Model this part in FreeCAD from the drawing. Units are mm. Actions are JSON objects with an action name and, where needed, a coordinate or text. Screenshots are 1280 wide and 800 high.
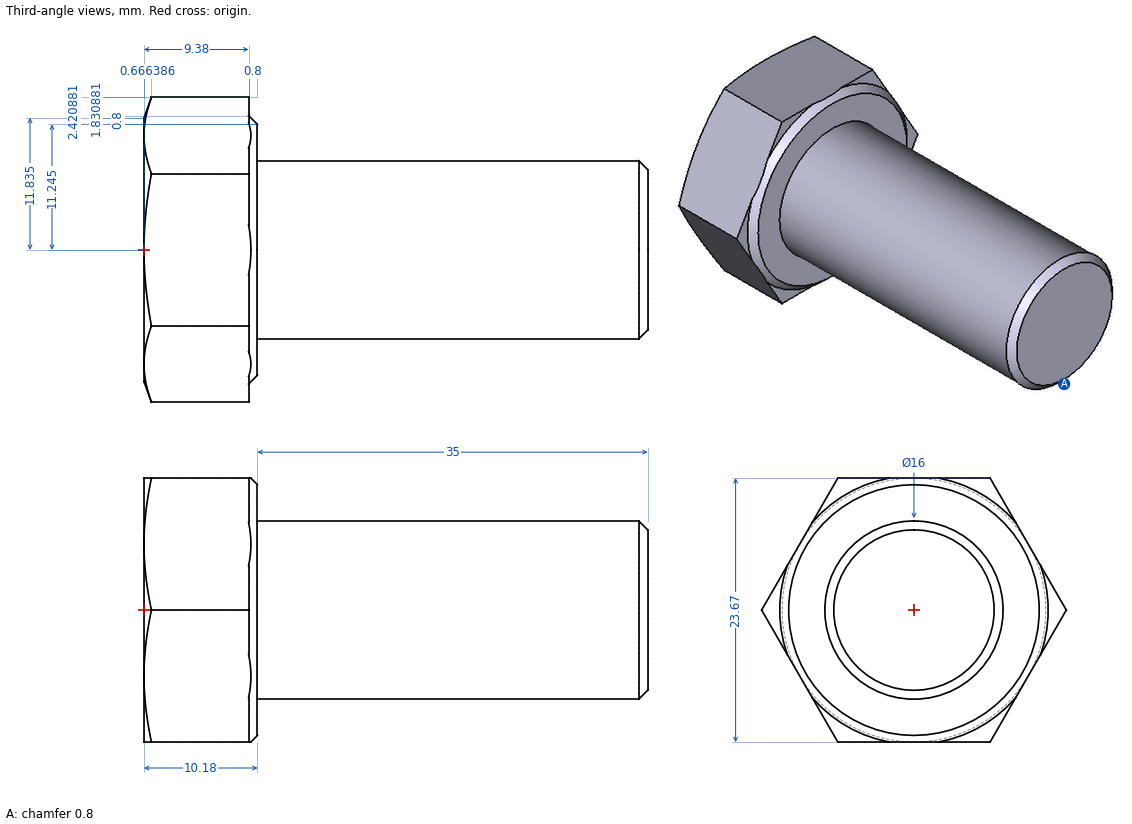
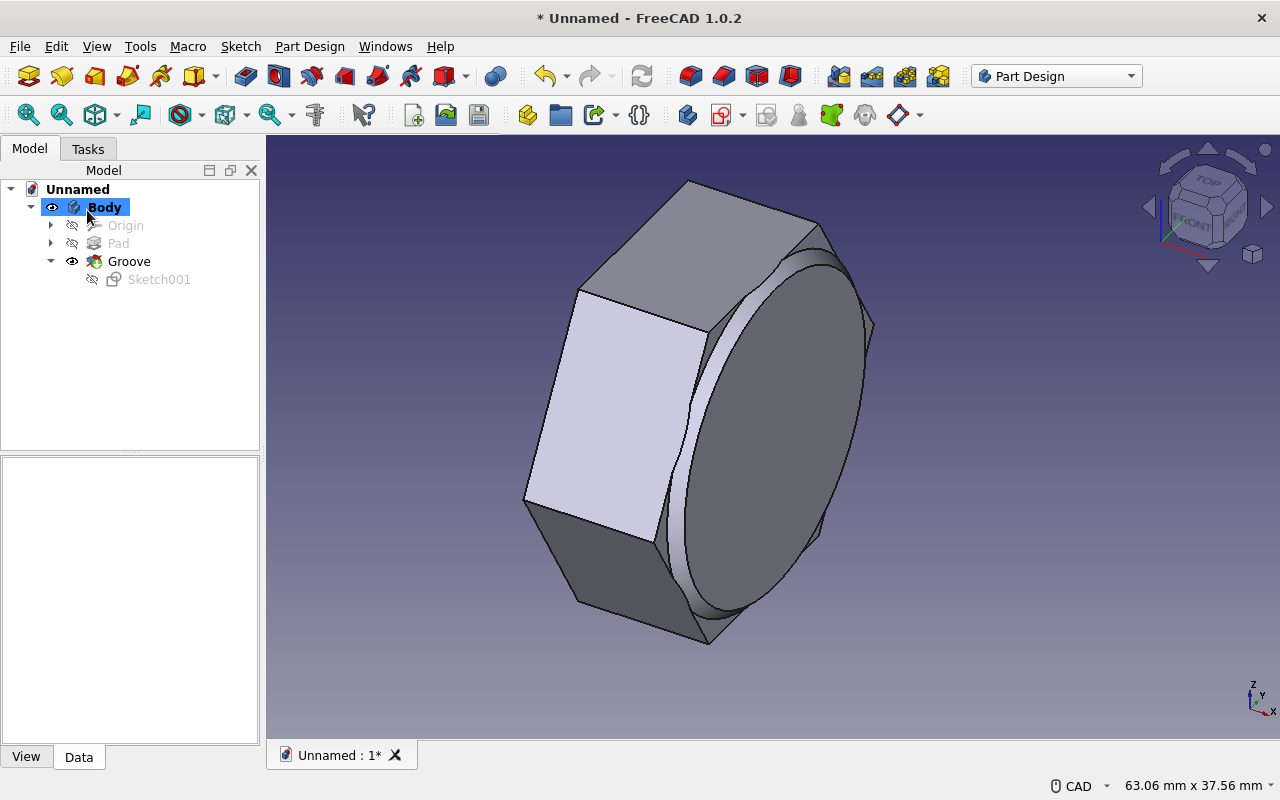
{"action": "key", "text": "v f"}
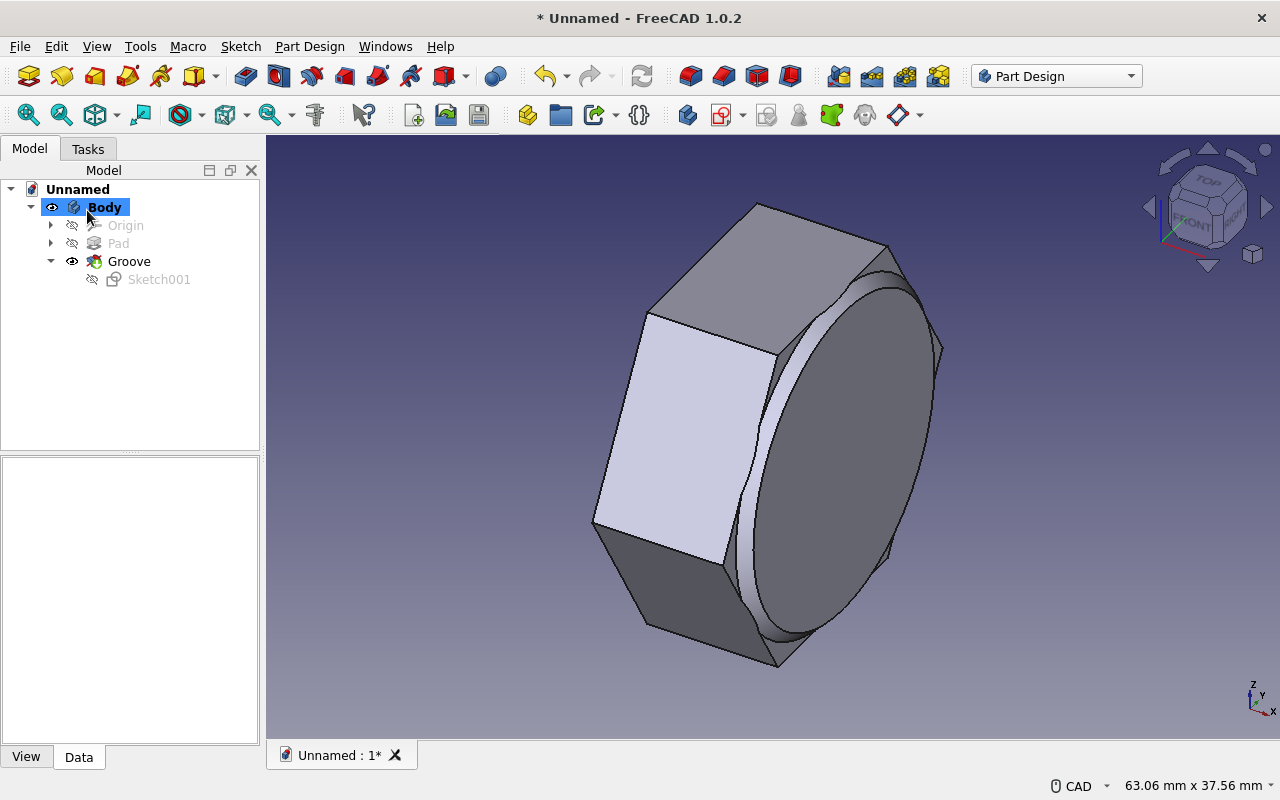
{"action": "left_click", "coordinate": [720, 116]}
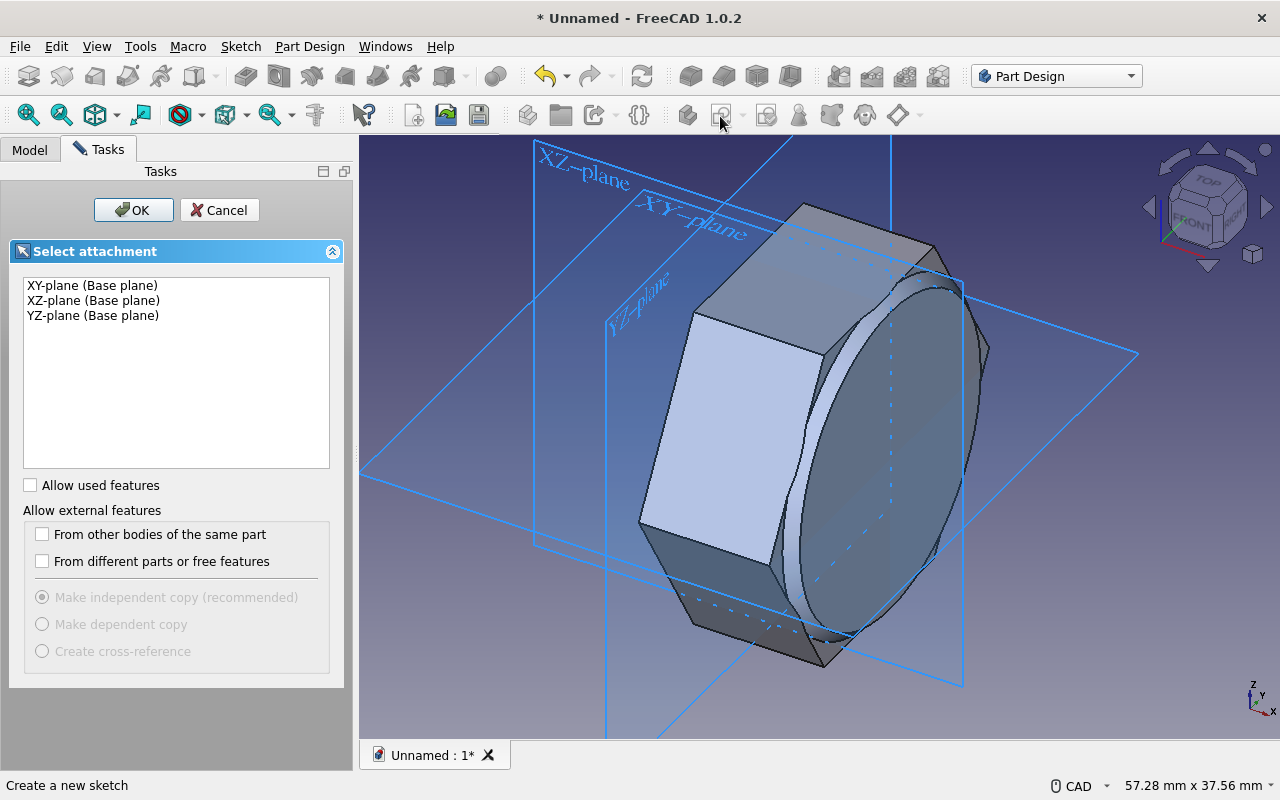
{"action": "left_click", "coordinate": [84, 286]}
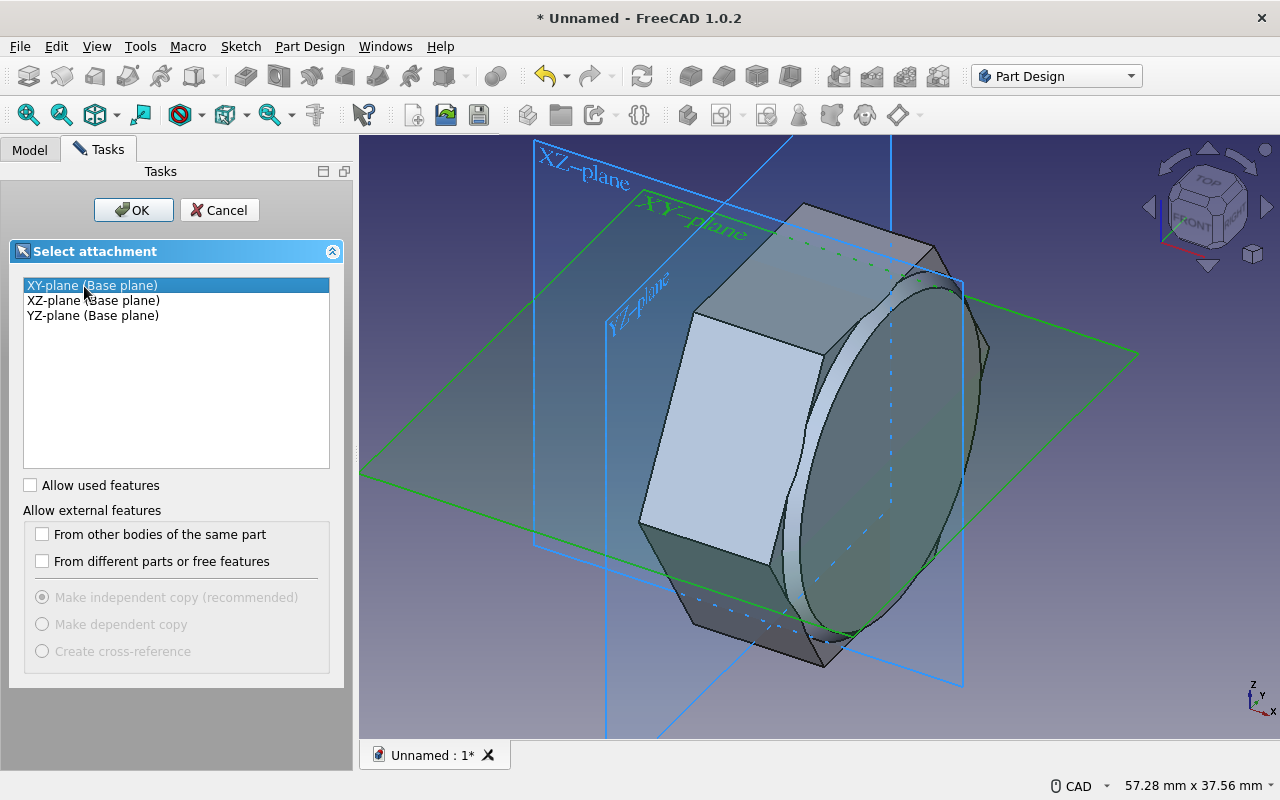
{"action": "left_click", "coordinate": [134, 210]}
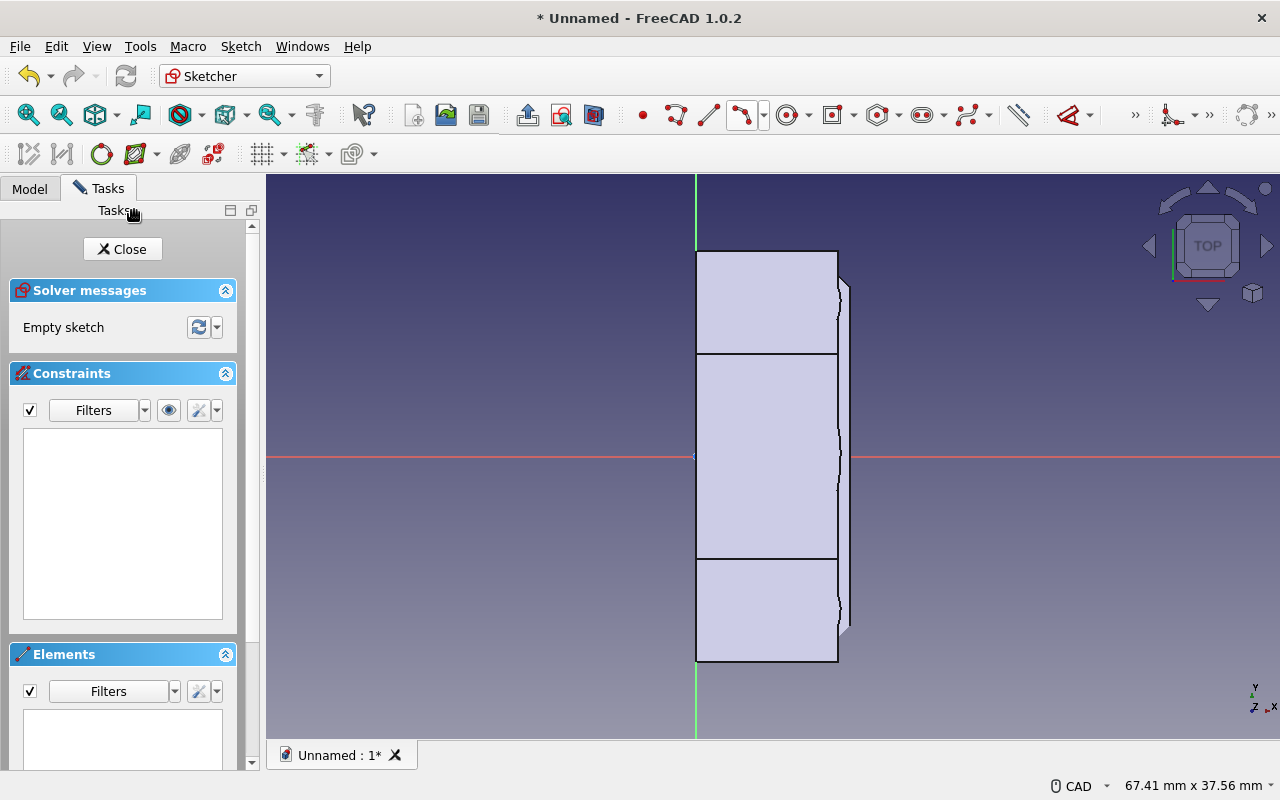
{"action": "left_click", "coordinate": [594, 116]}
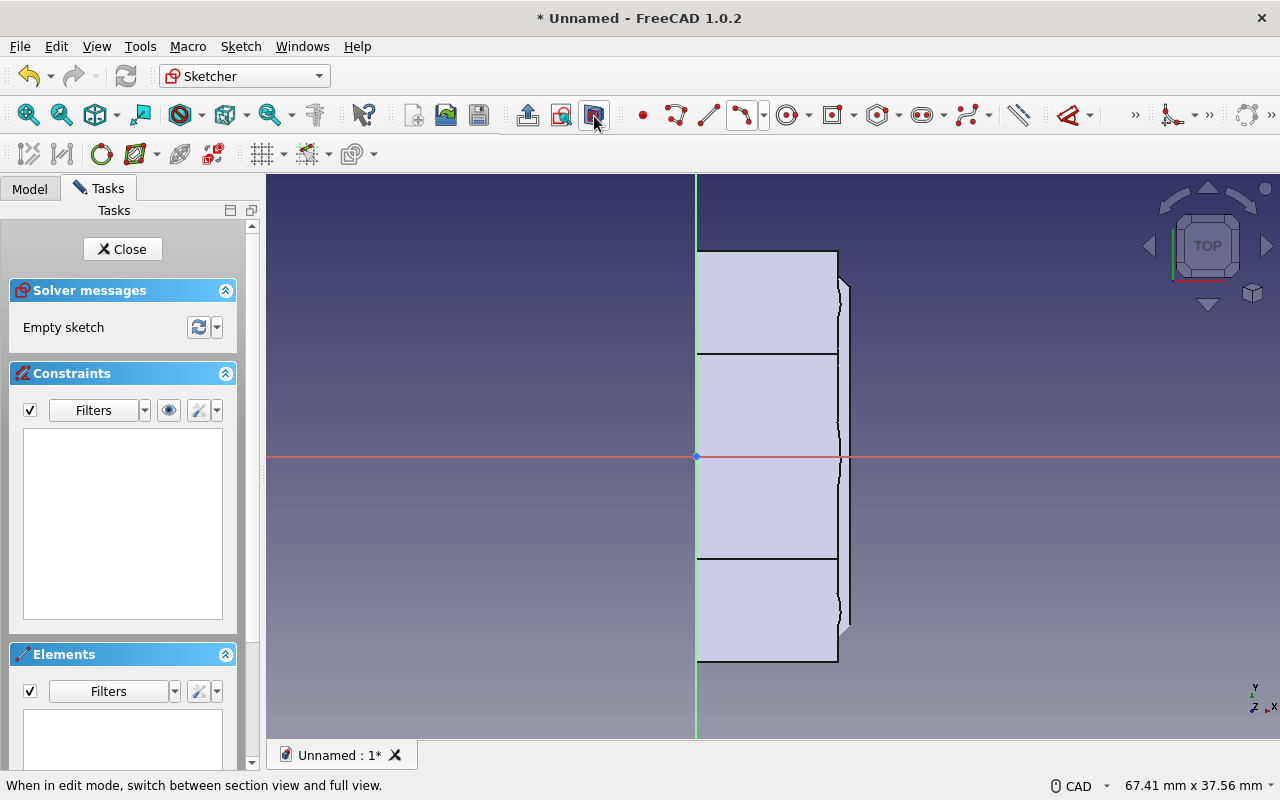
{"action": "scroll", "coordinate": [701, 249], "scroll_direction": "up", "scroll_amount": 13}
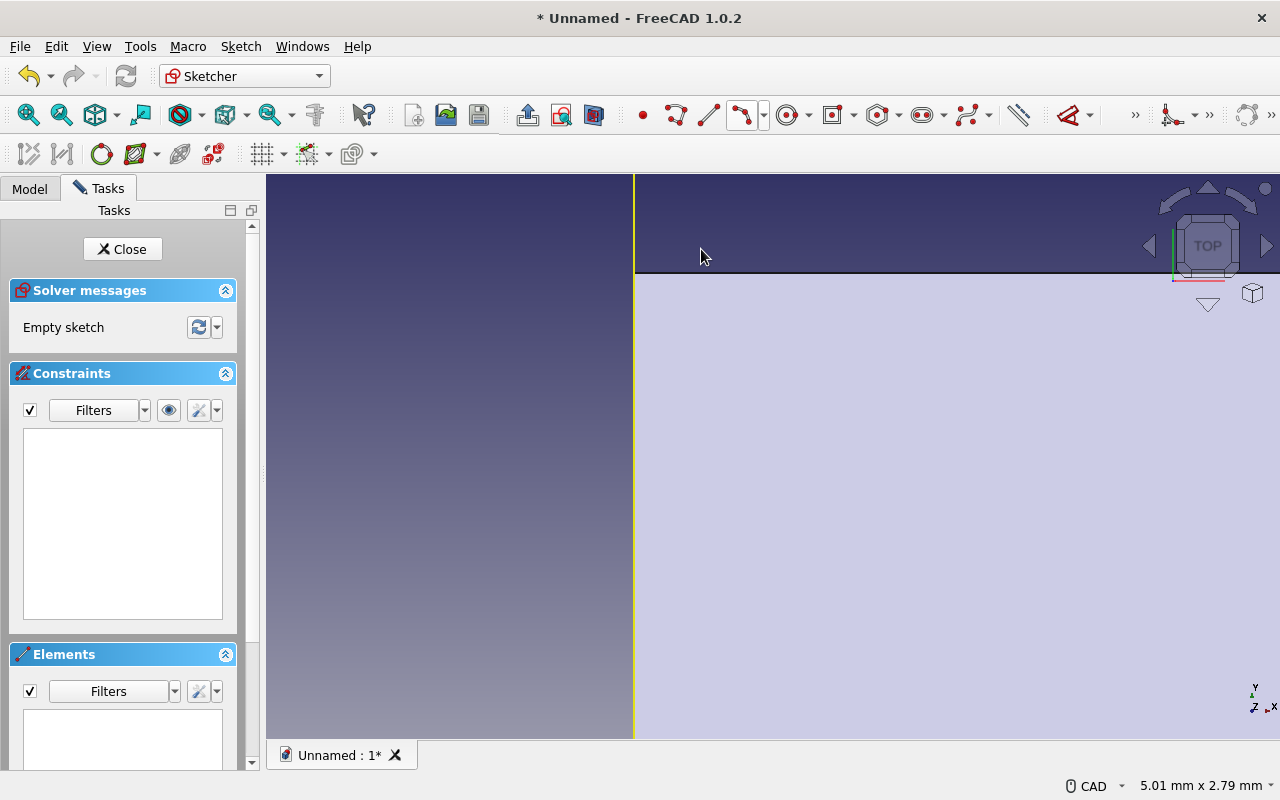
{"action": "left_click", "coordinate": [676, 116]}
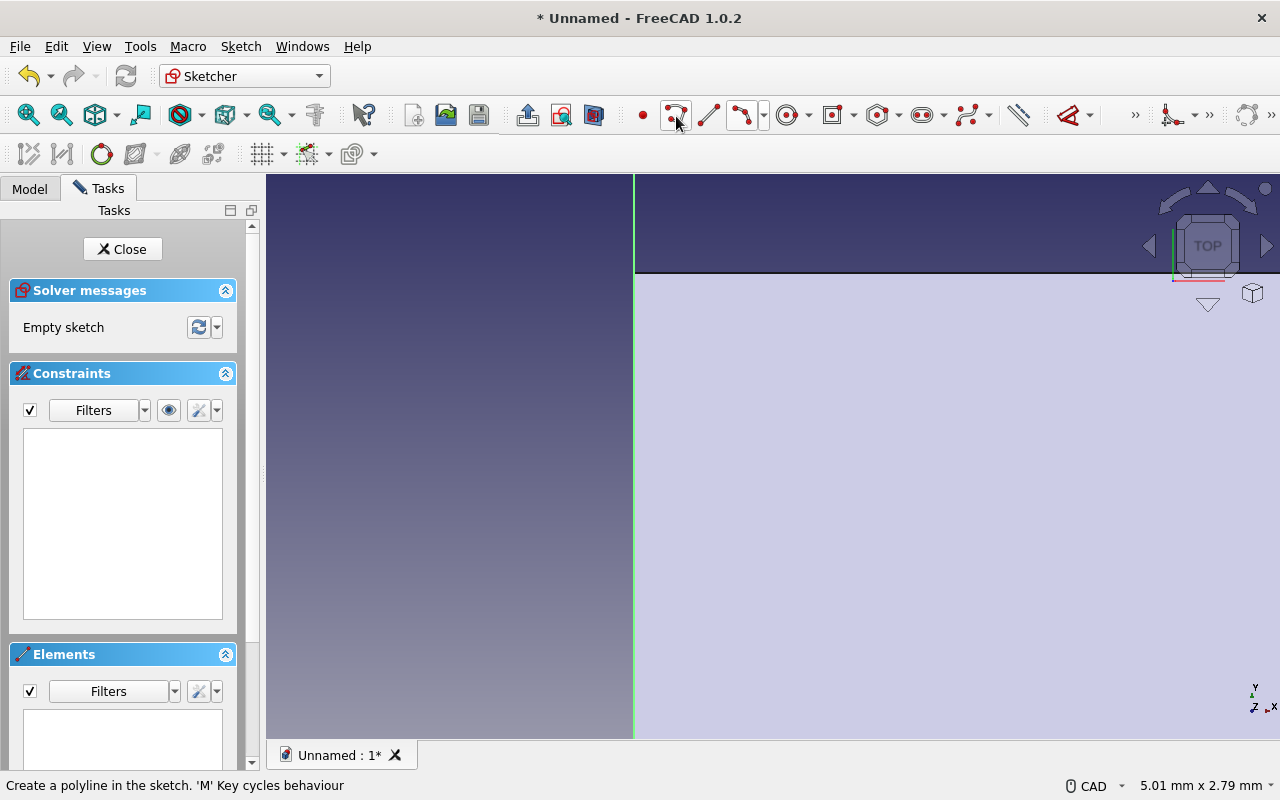
{"action": "left_click", "coordinate": [634, 644]}
{"action": "left_click", "coordinate": [769, 273]}
{"action": "left_click", "coordinate": [643, 273]}
{"action": "left_click", "coordinate": [634, 645]}
{"action": "key", "text": "Escape"}
{"action": "key", "text": "Escape"}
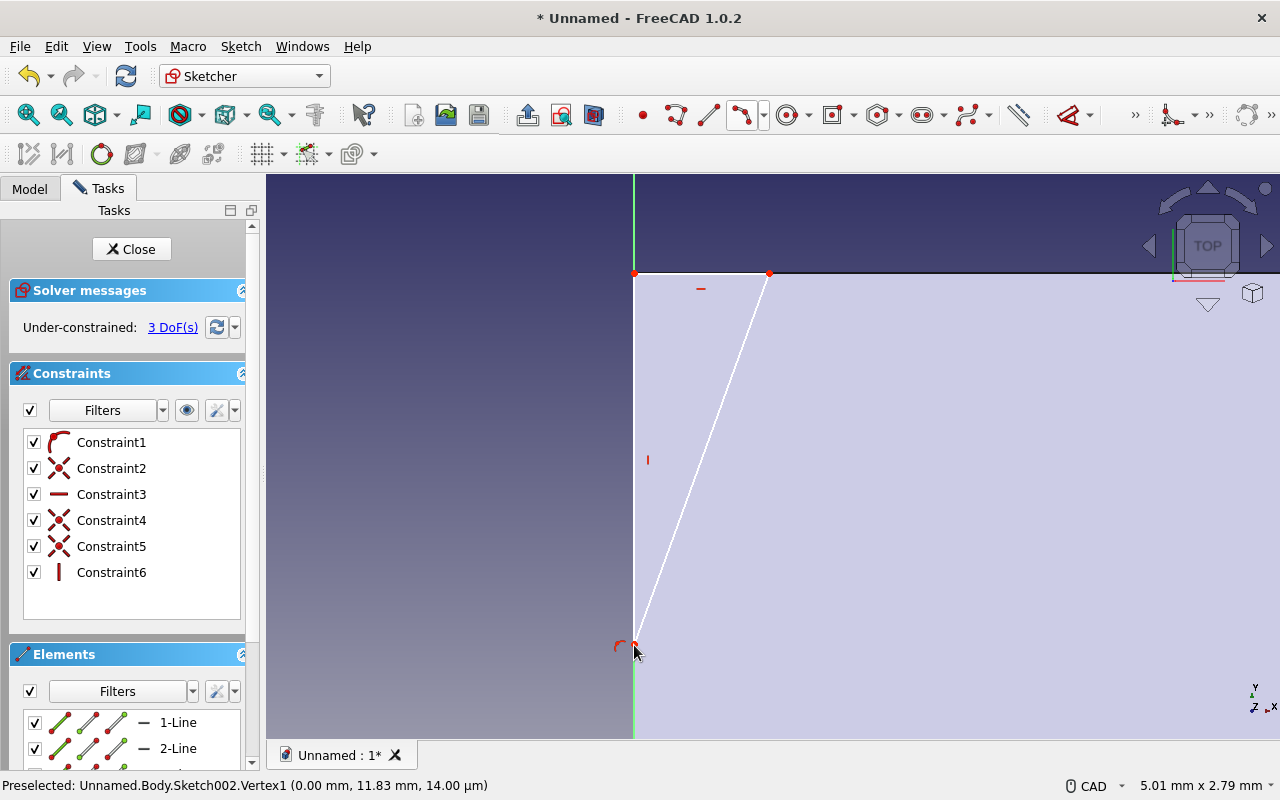
{"action": "left_click", "coordinate": [1068, 116]}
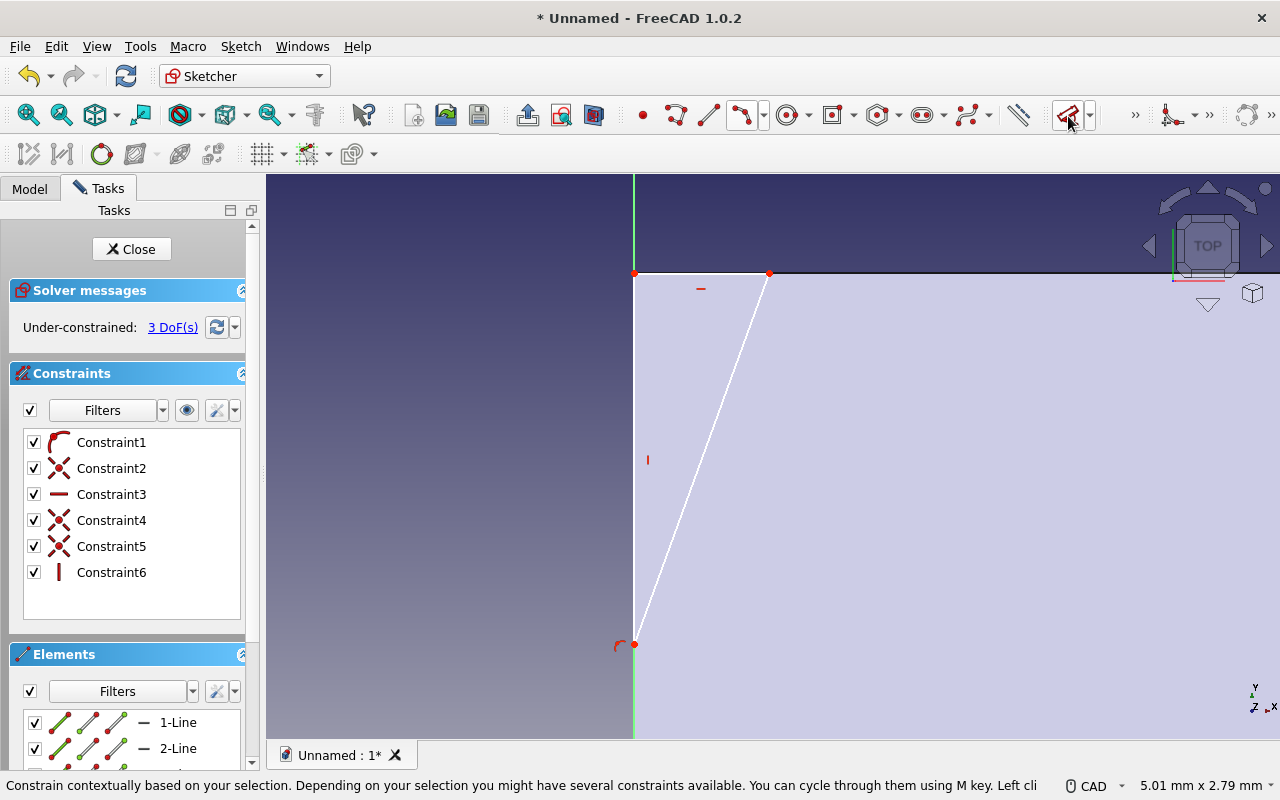
{"action": "left_click", "coordinate": [634, 645]}
{"action": "left_click", "coordinate": [600, 678]}